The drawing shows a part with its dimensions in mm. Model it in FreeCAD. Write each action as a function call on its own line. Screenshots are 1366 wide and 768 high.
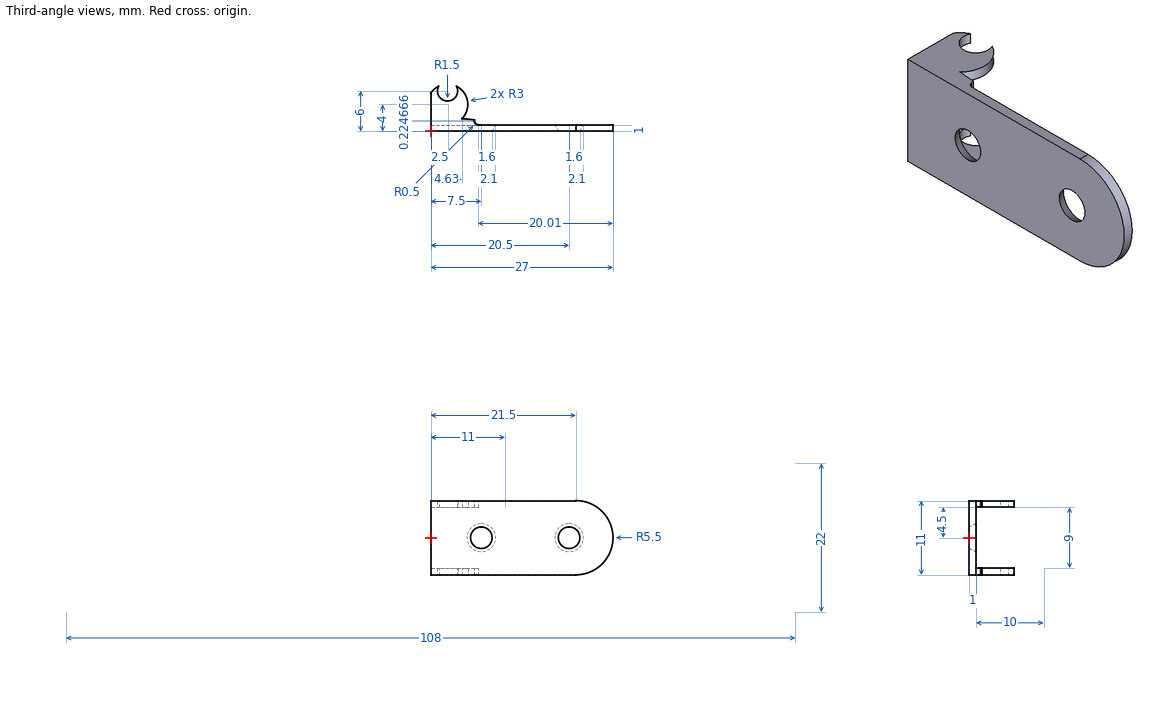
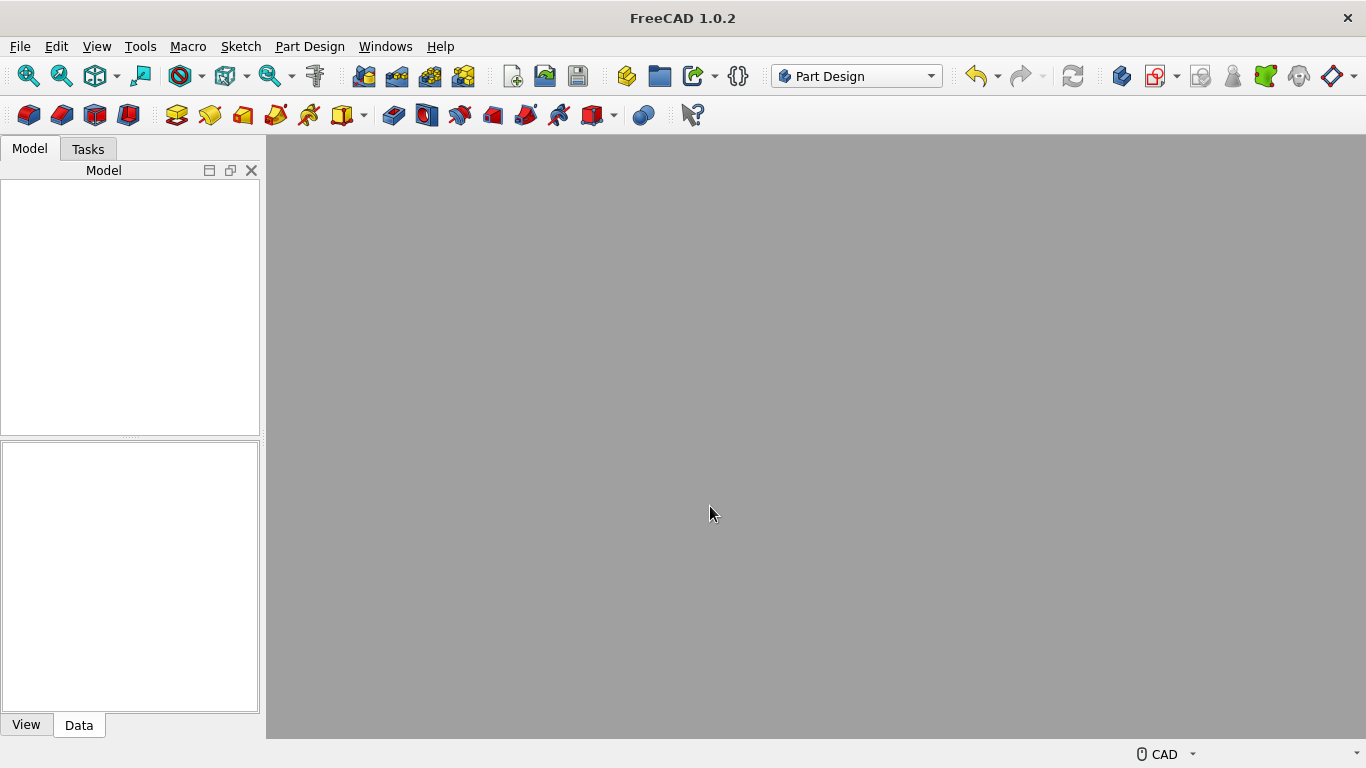
key(ctrl+n)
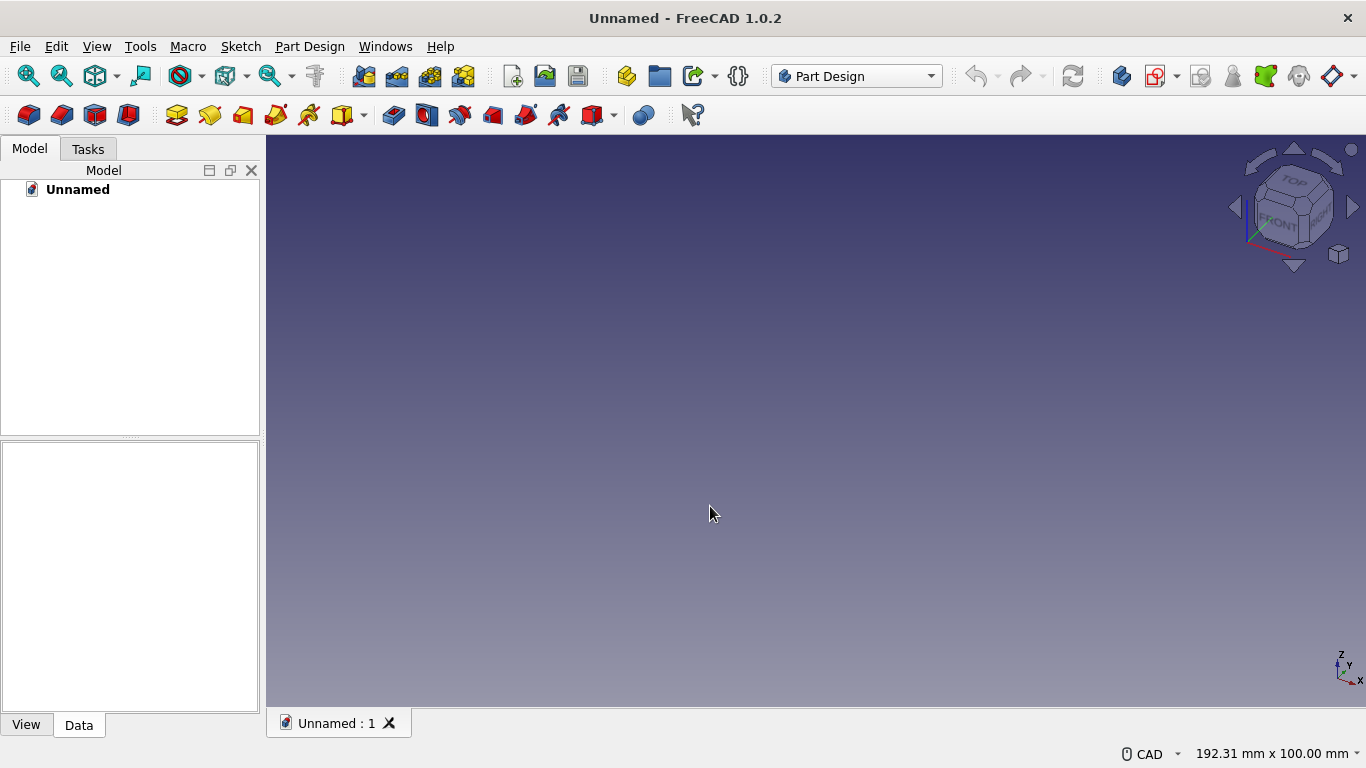
click(1154, 76)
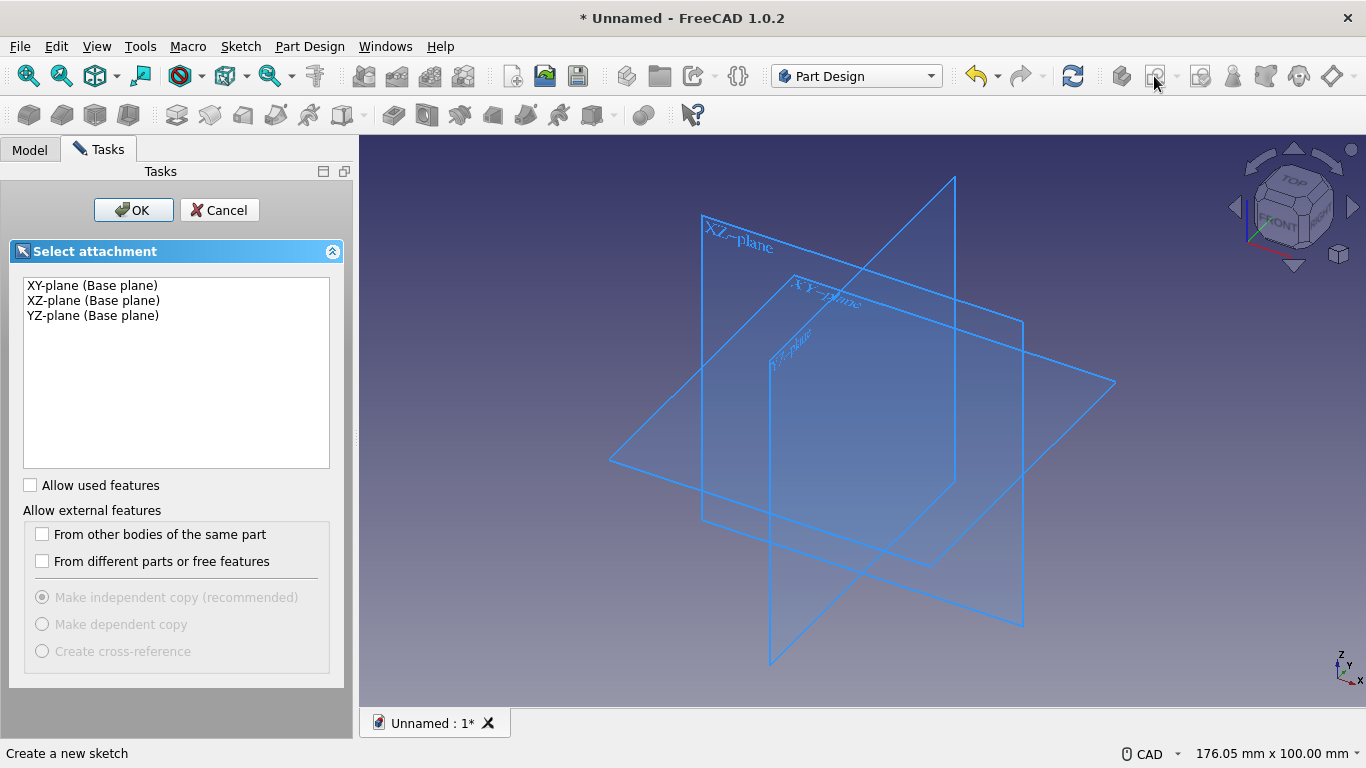
click(84, 286)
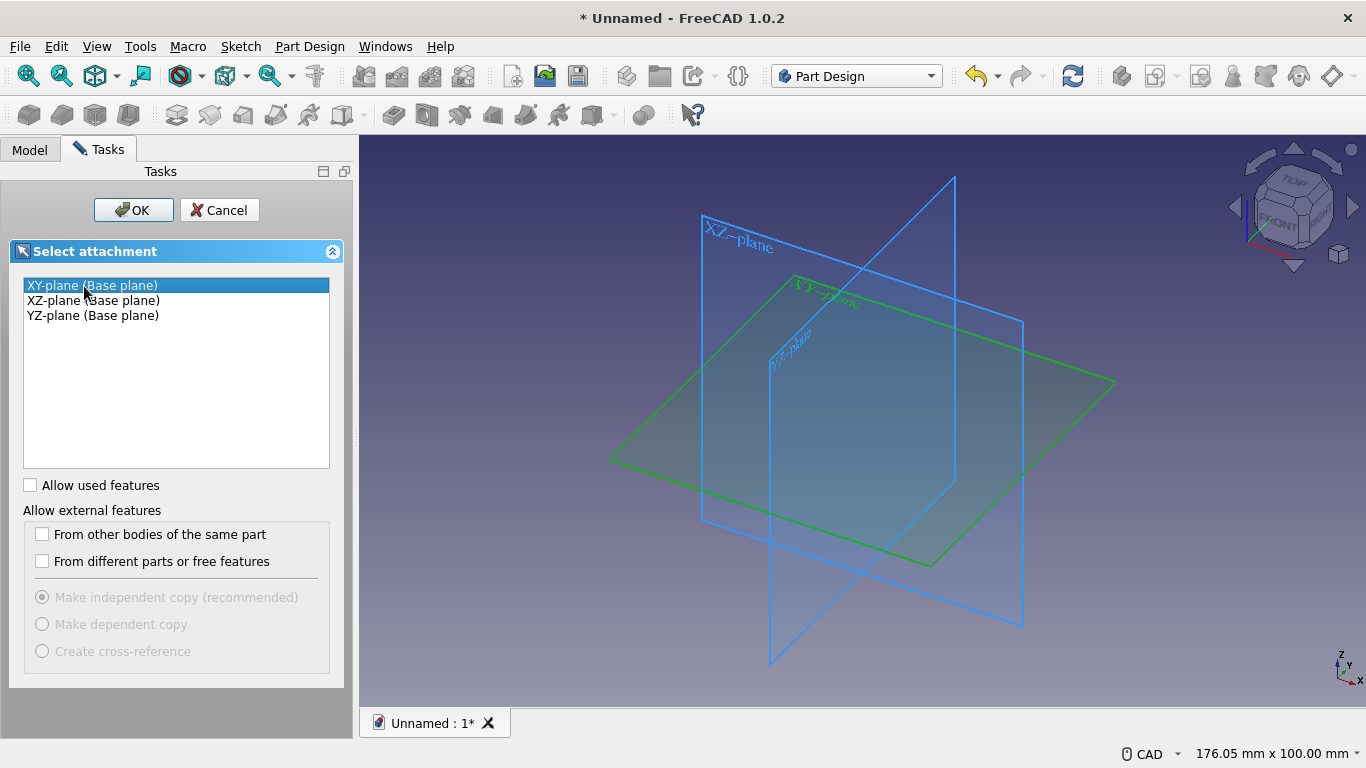
click(134, 210)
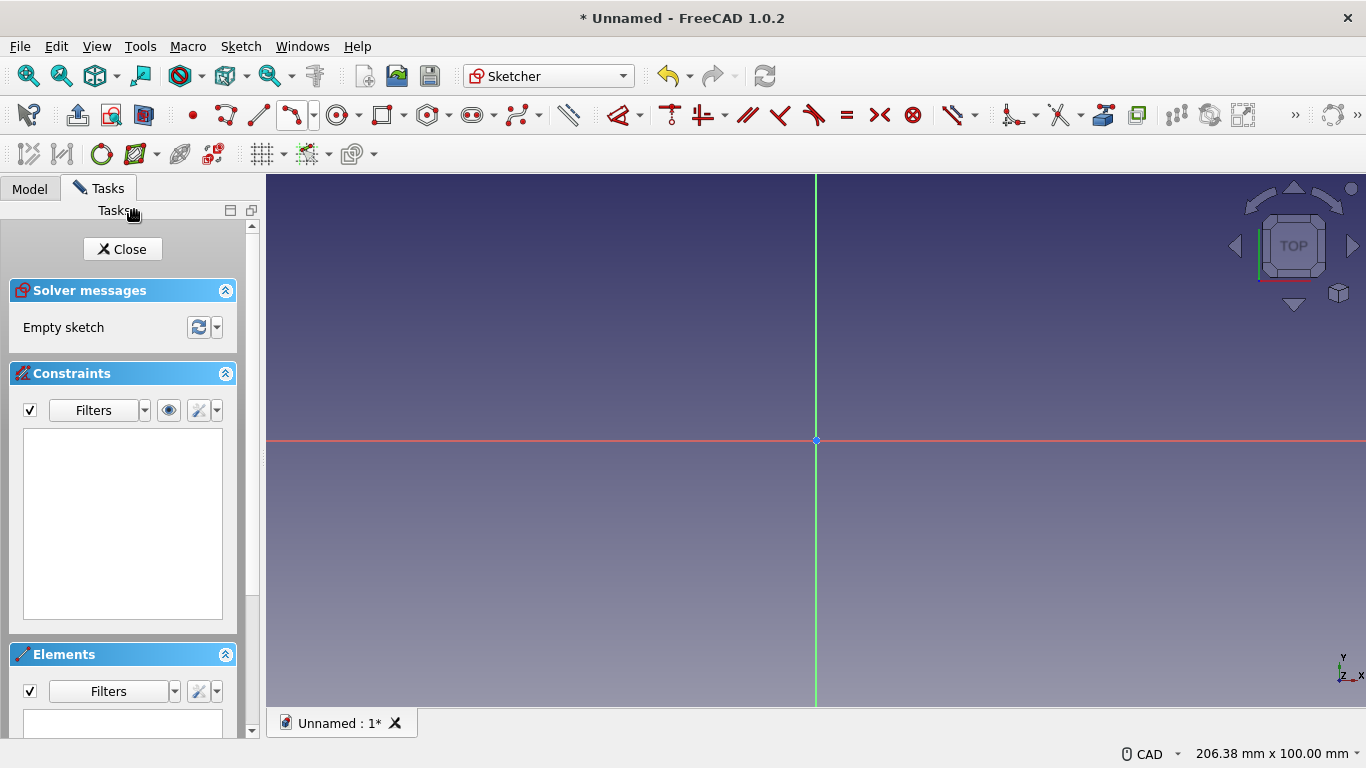
scroll(934, 417, up, 7)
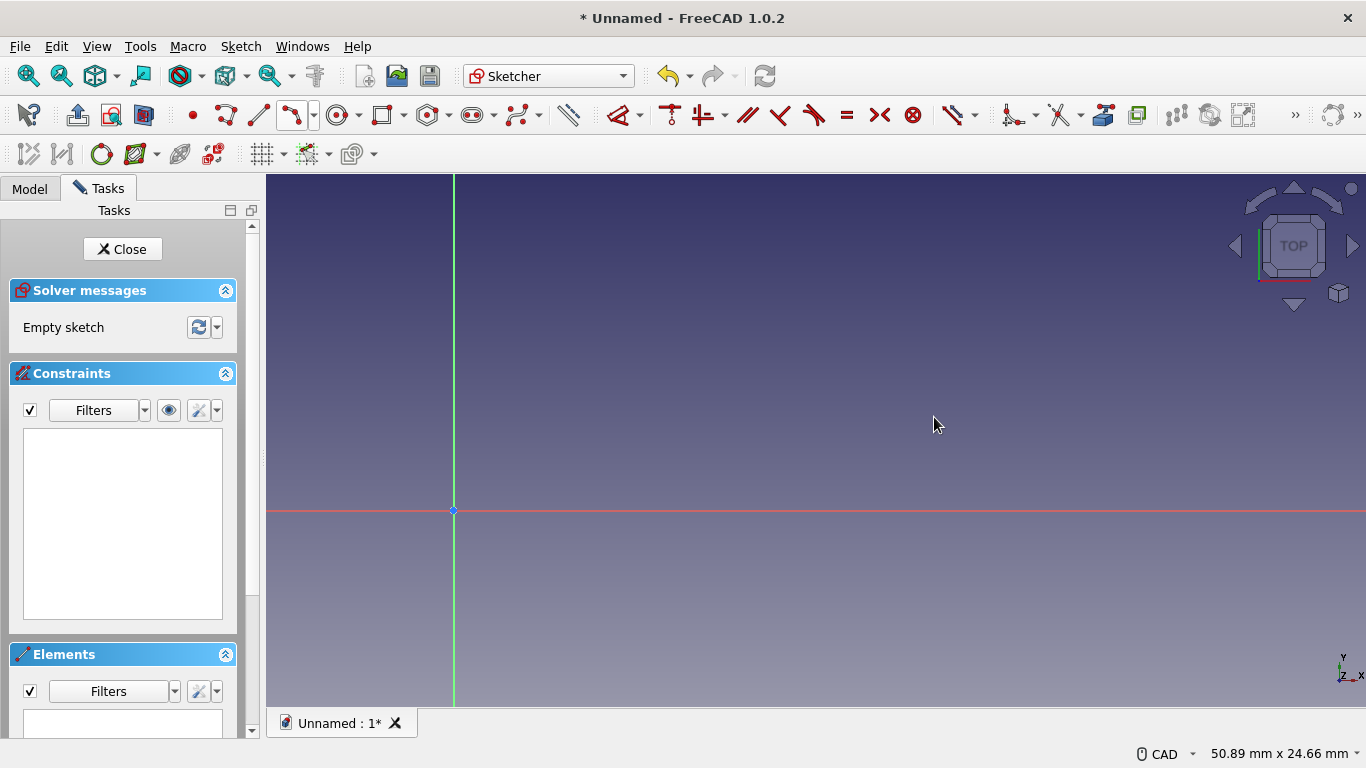
key(g)
key(m)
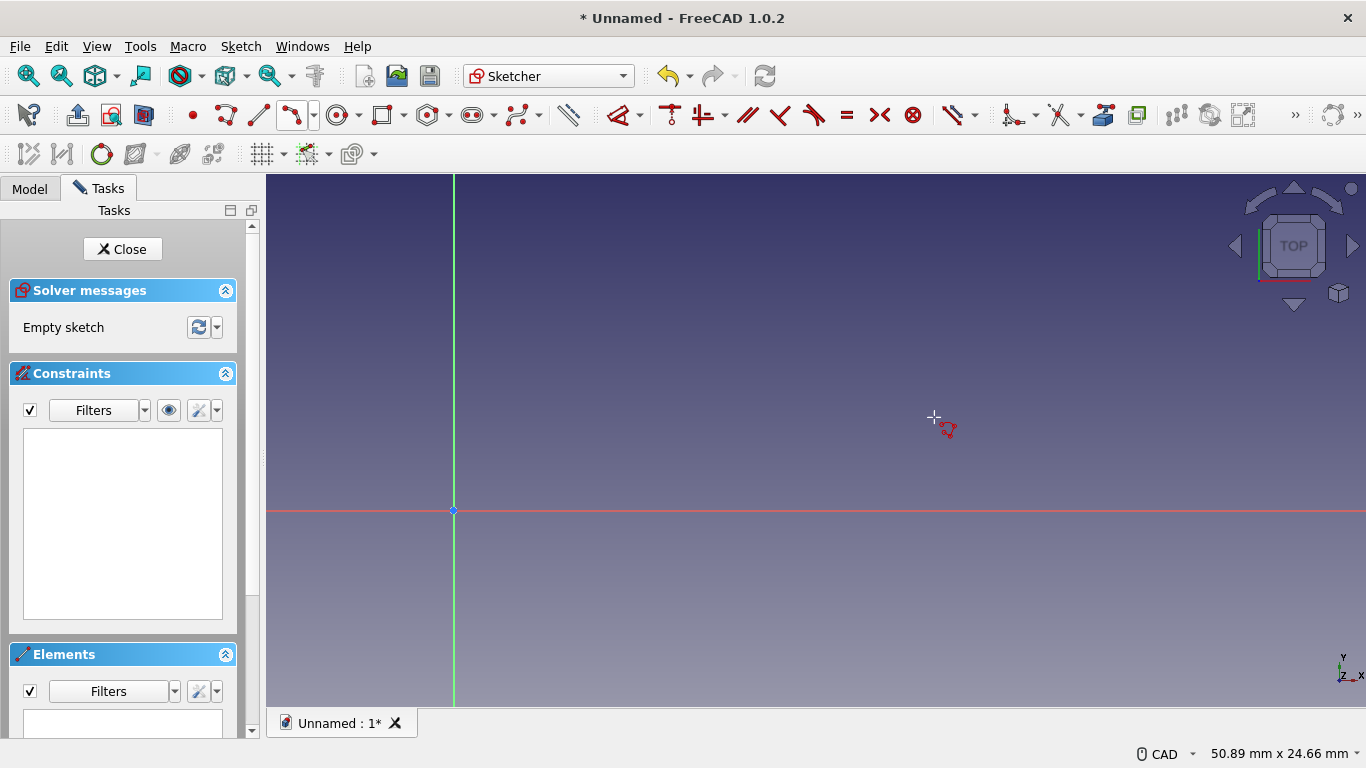
click(594, 478)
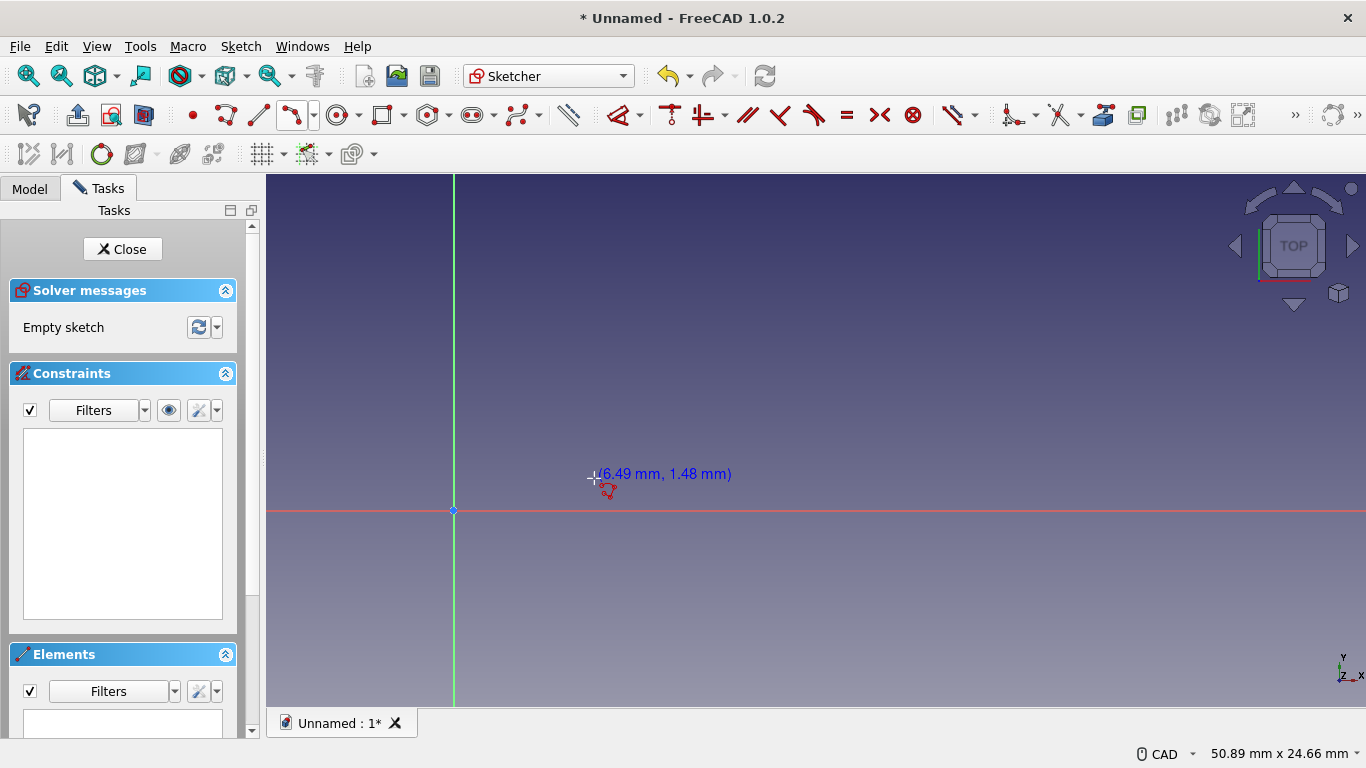
scroll(594, 474, up, 6)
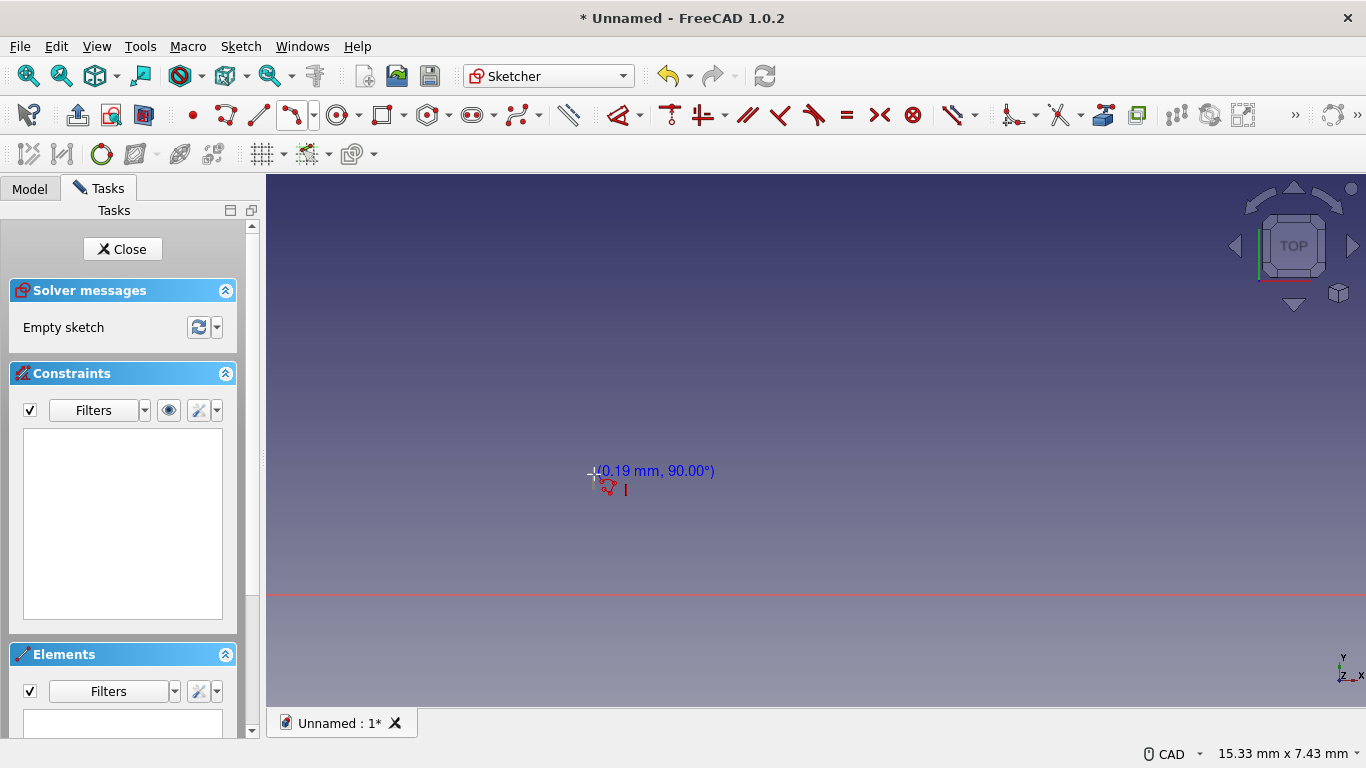
click(593, 471)
click(460, 460)
right_click(460, 460)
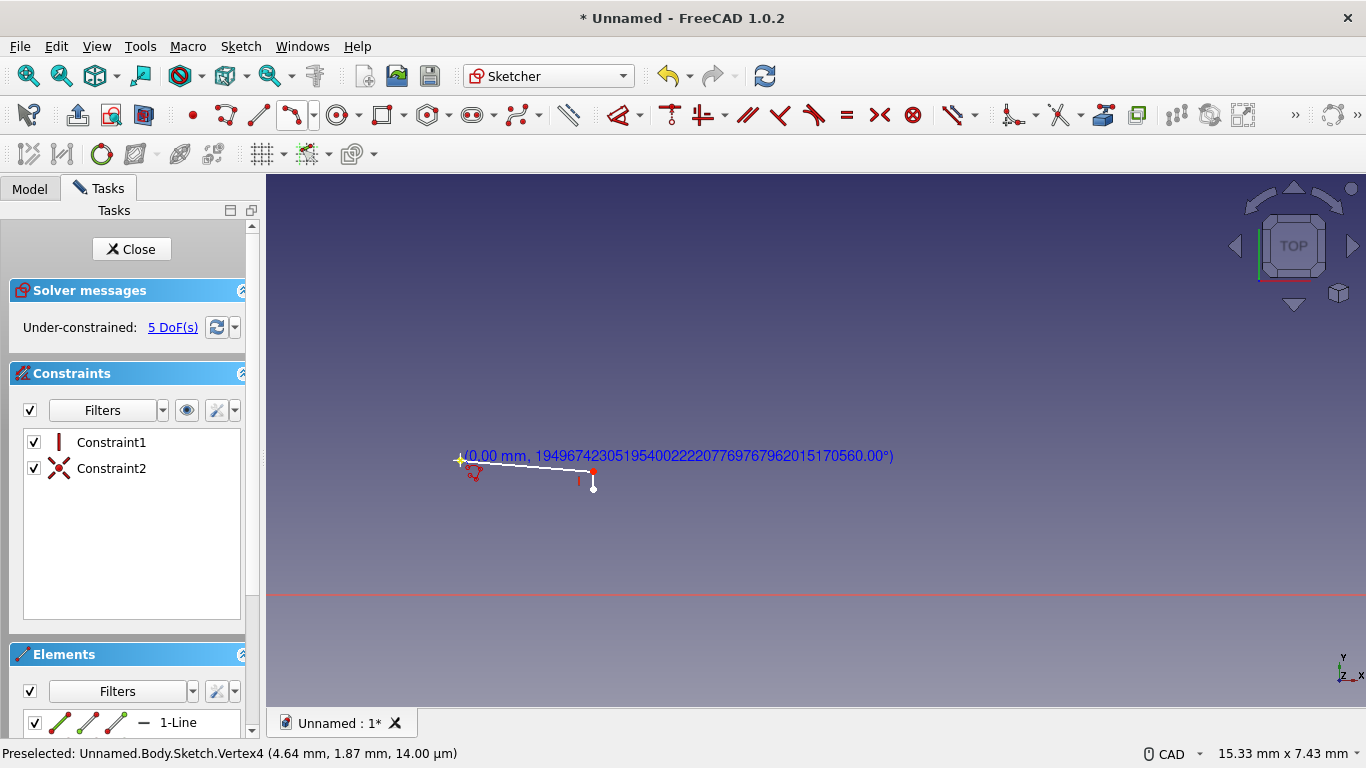
scroll(597, 477, down, 6)